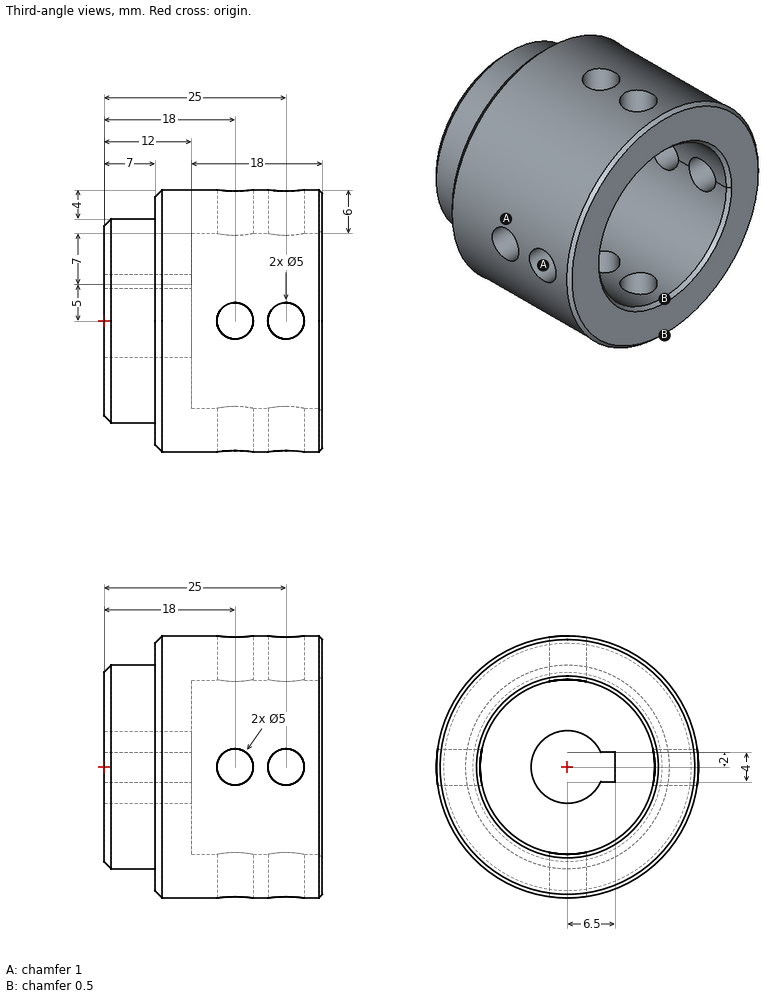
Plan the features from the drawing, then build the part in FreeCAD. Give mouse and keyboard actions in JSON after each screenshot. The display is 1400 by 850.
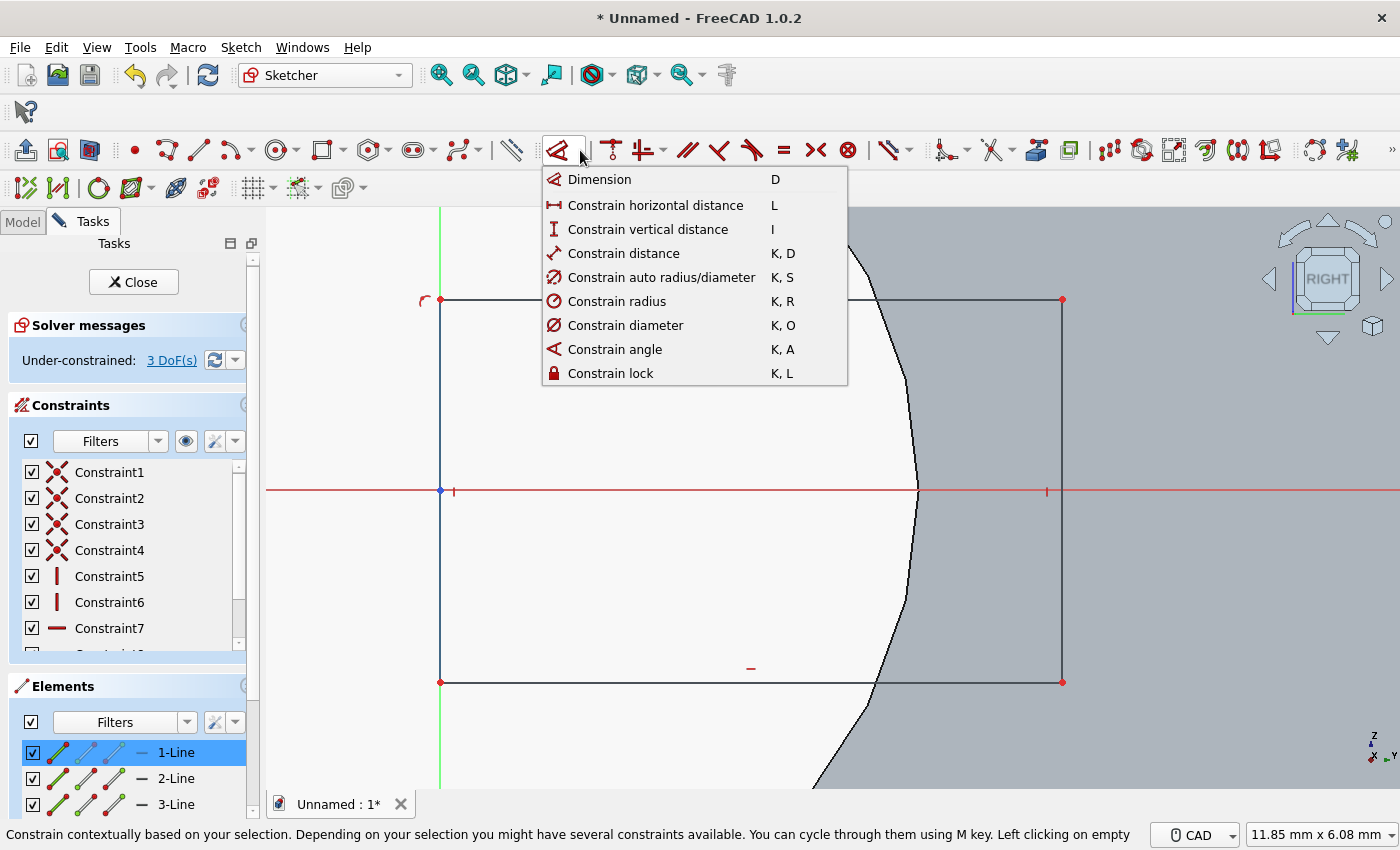
{"action": "left_click", "coordinate": [695, 229]}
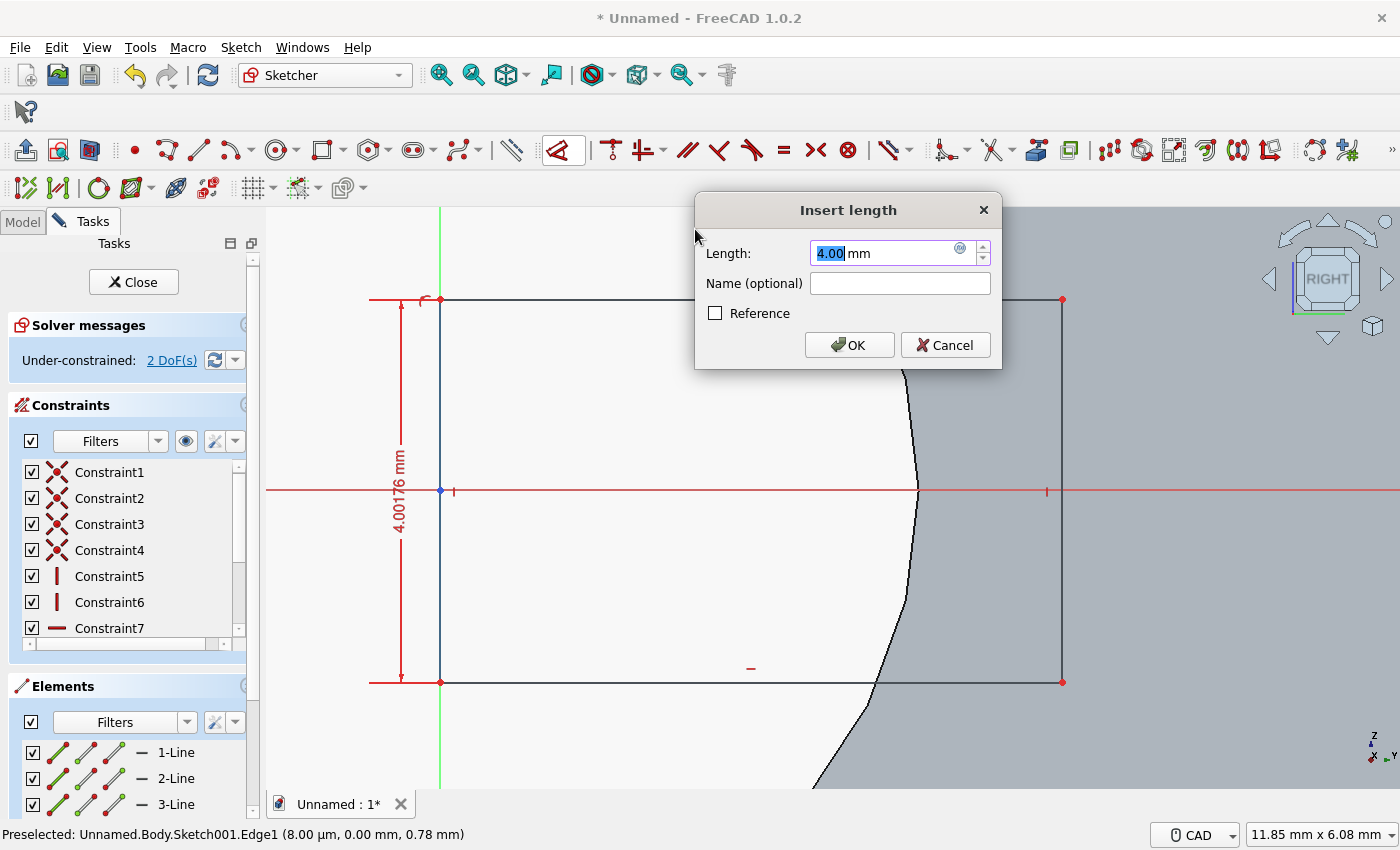
{"action": "type", "text": "4"}
{"action": "key", "text": "Return"}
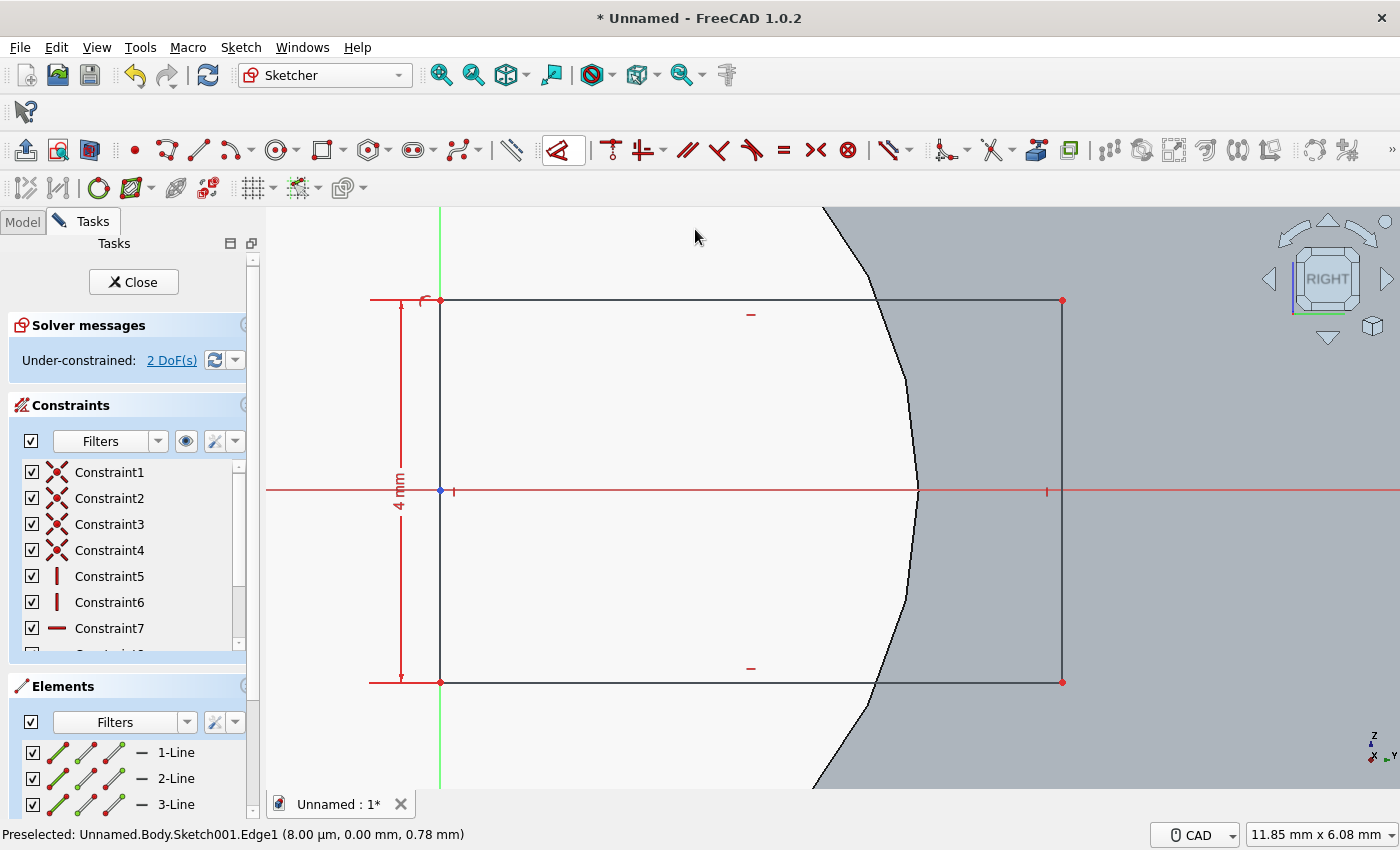
{"action": "left_click", "coordinate": [440, 300]}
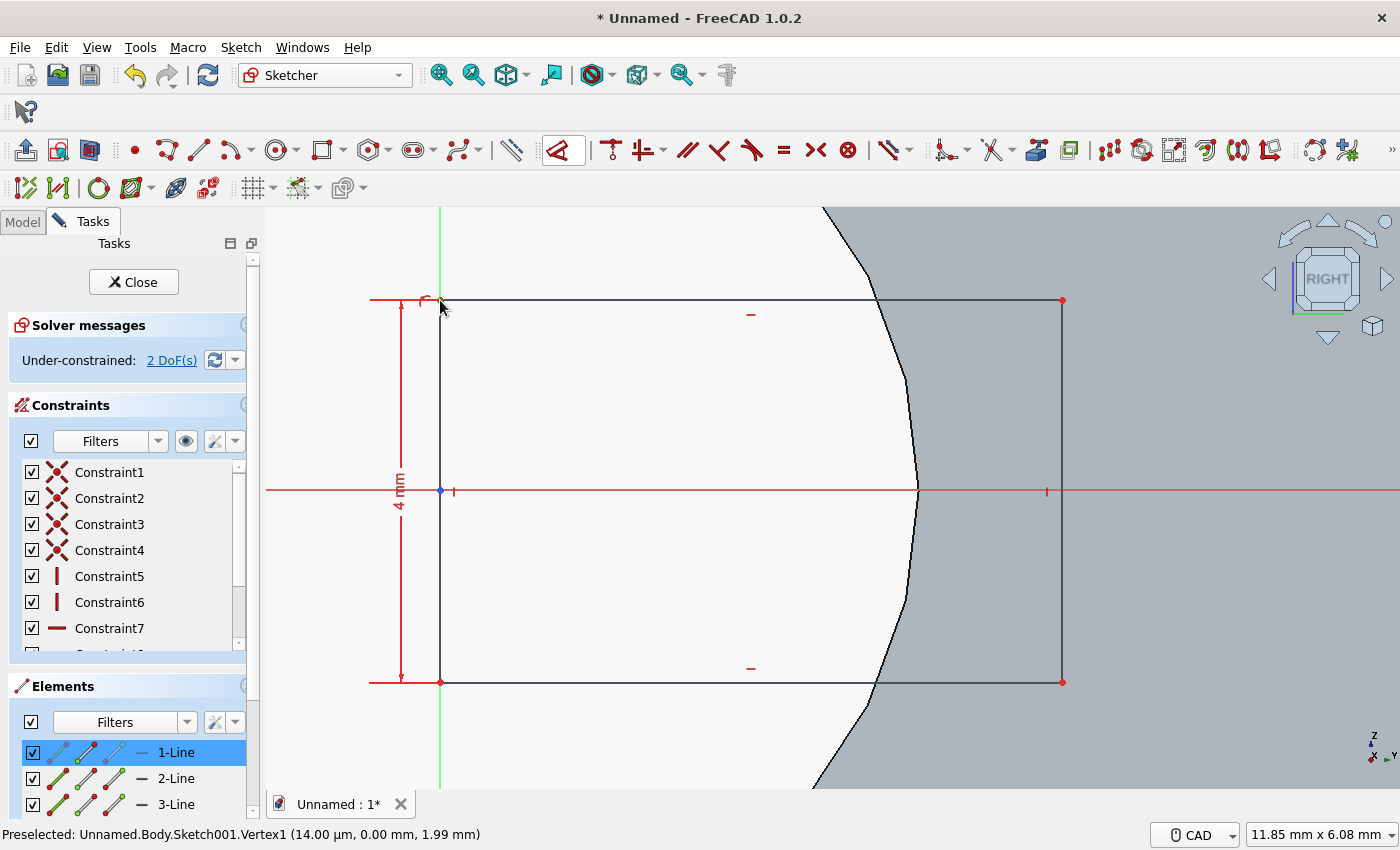
{"action": "left_click", "coordinate": [580, 150]}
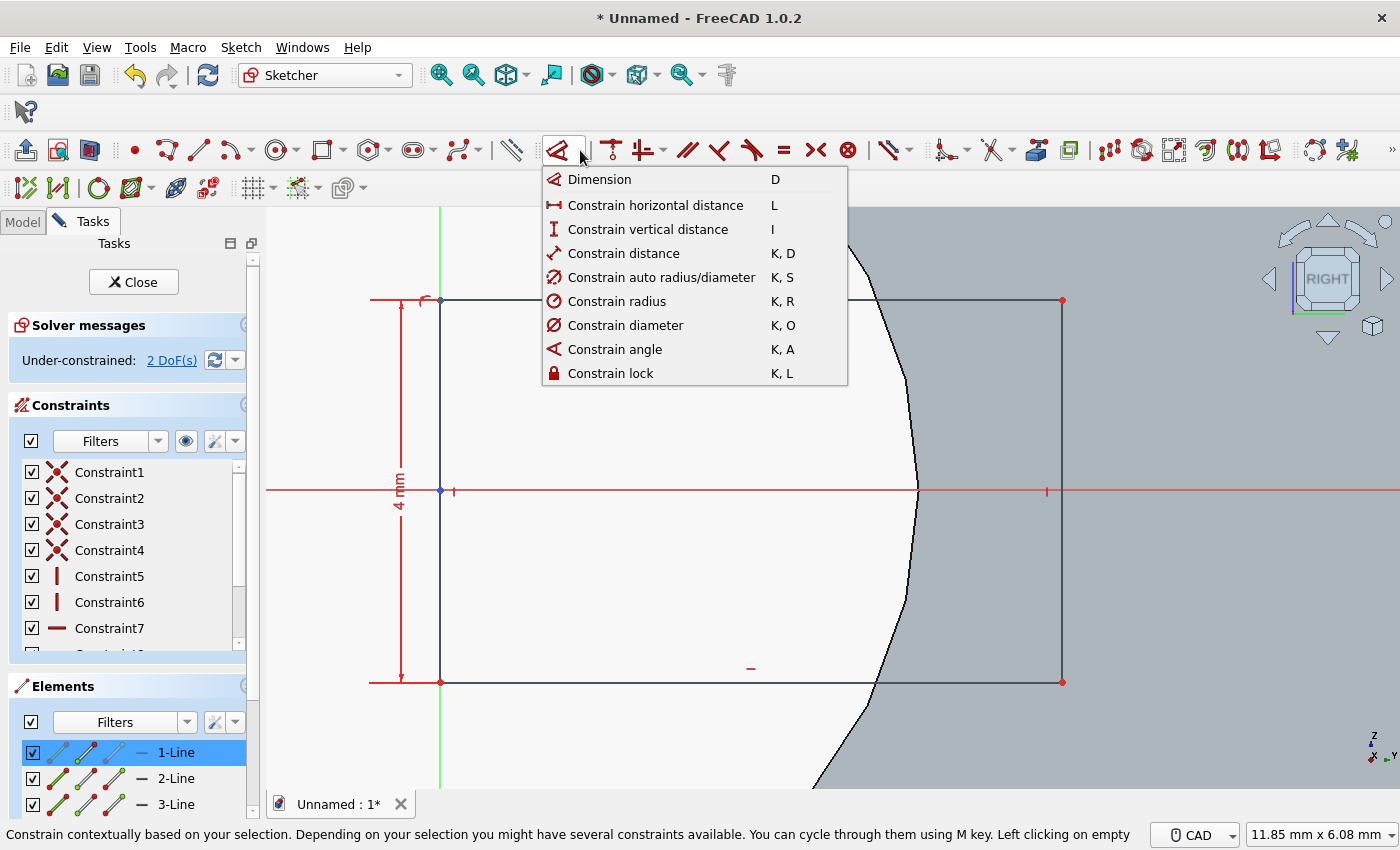
{"action": "left_click", "coordinate": [695, 229]}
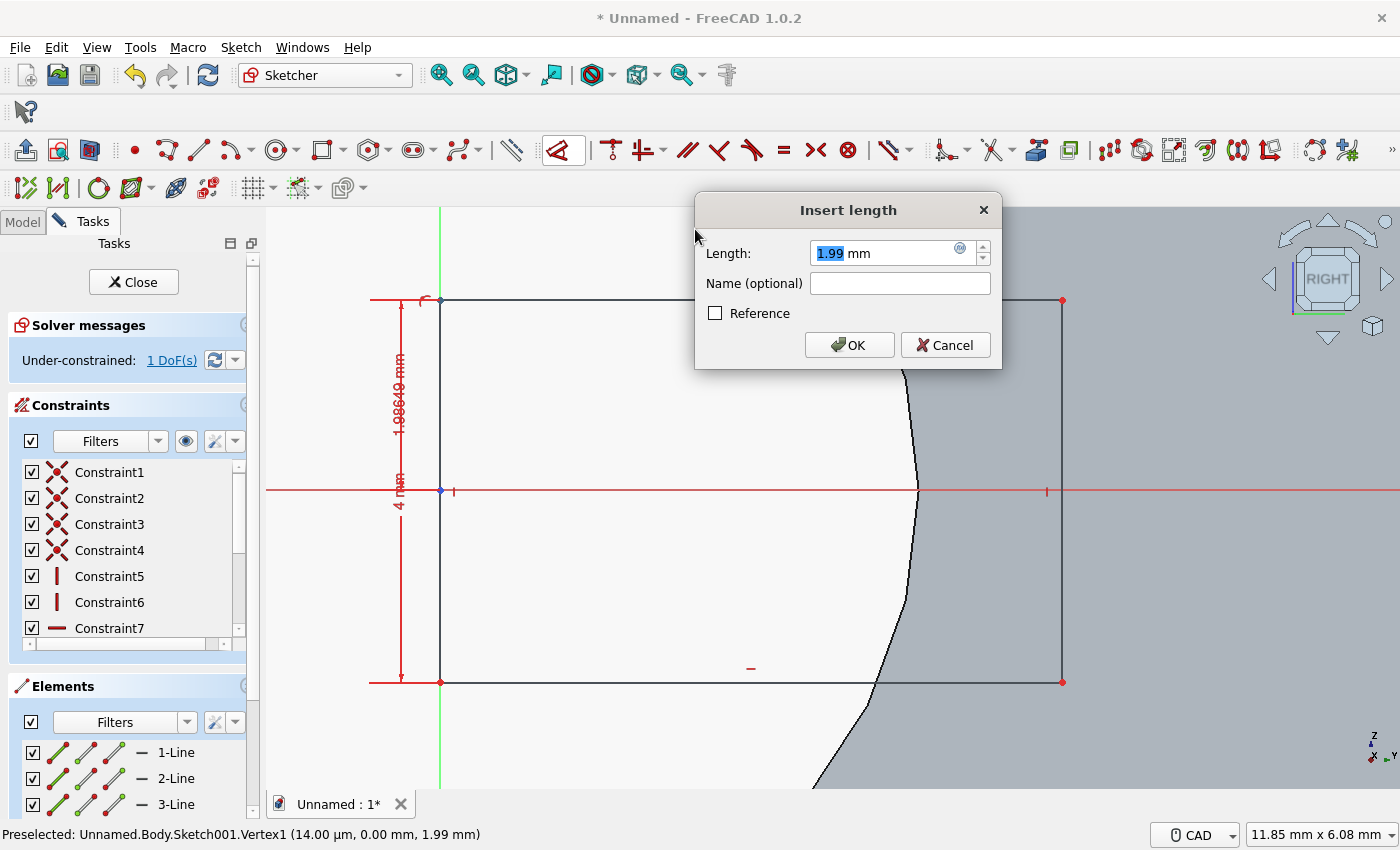
{"action": "type", "text": "2"}
{"action": "key", "text": "Return"}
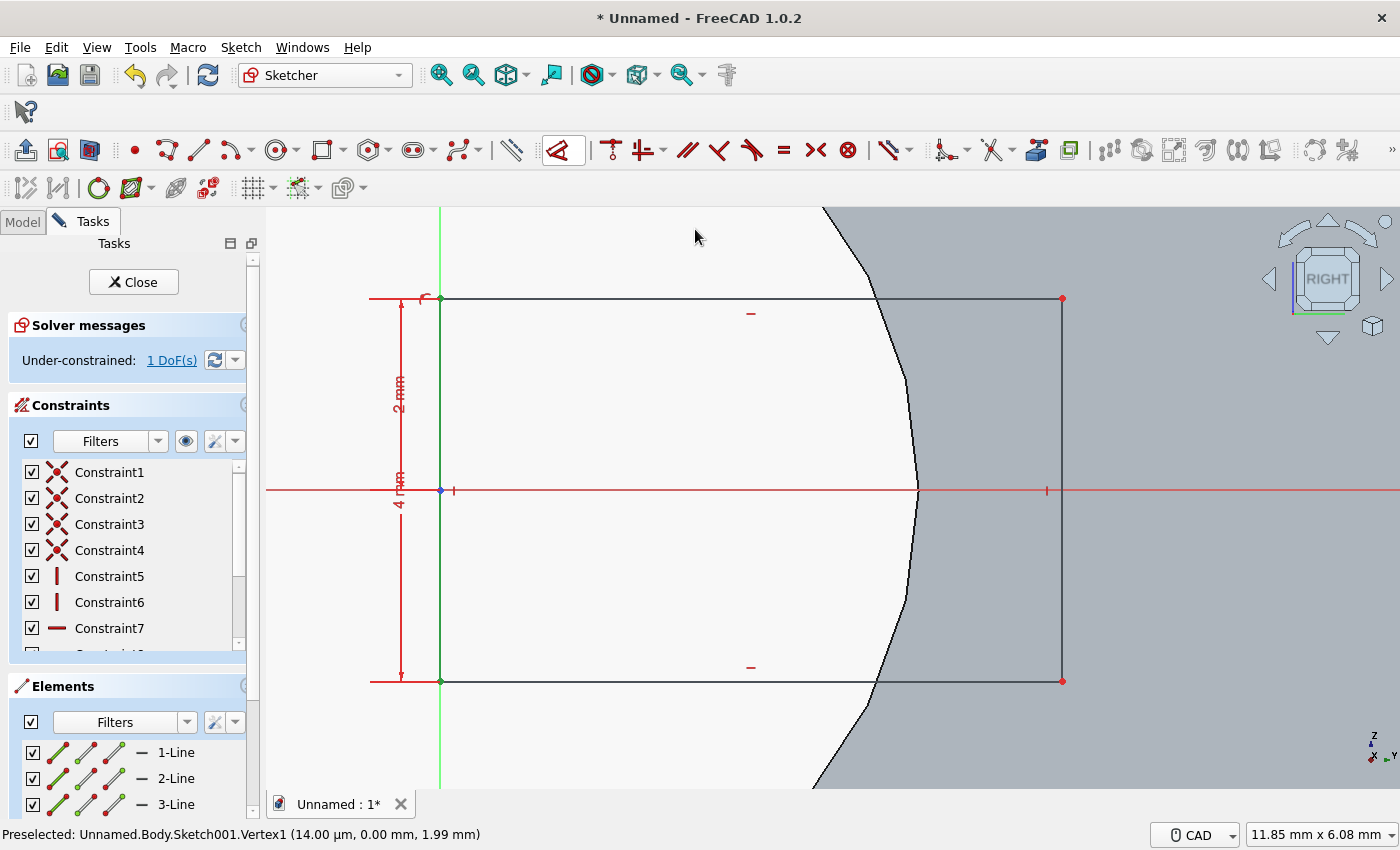
{"action": "left_click", "coordinate": [627, 682]}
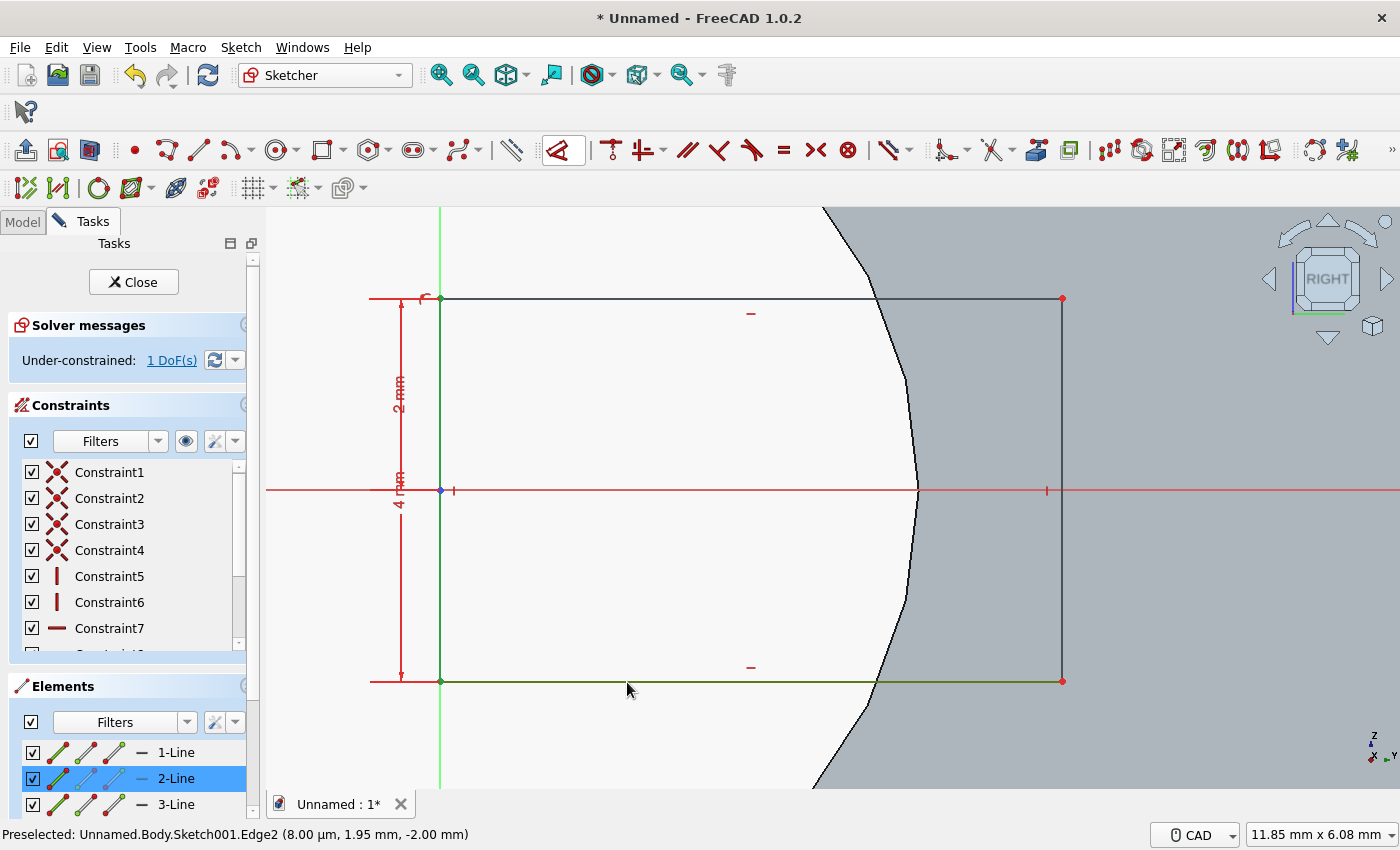
{"action": "key", "text": "l"}